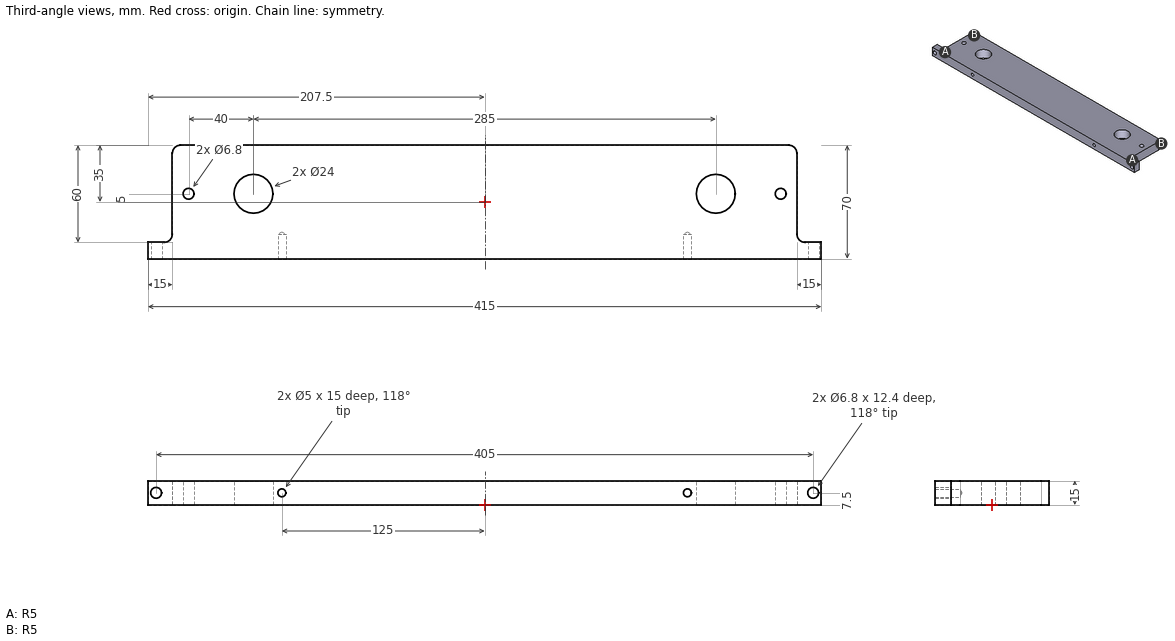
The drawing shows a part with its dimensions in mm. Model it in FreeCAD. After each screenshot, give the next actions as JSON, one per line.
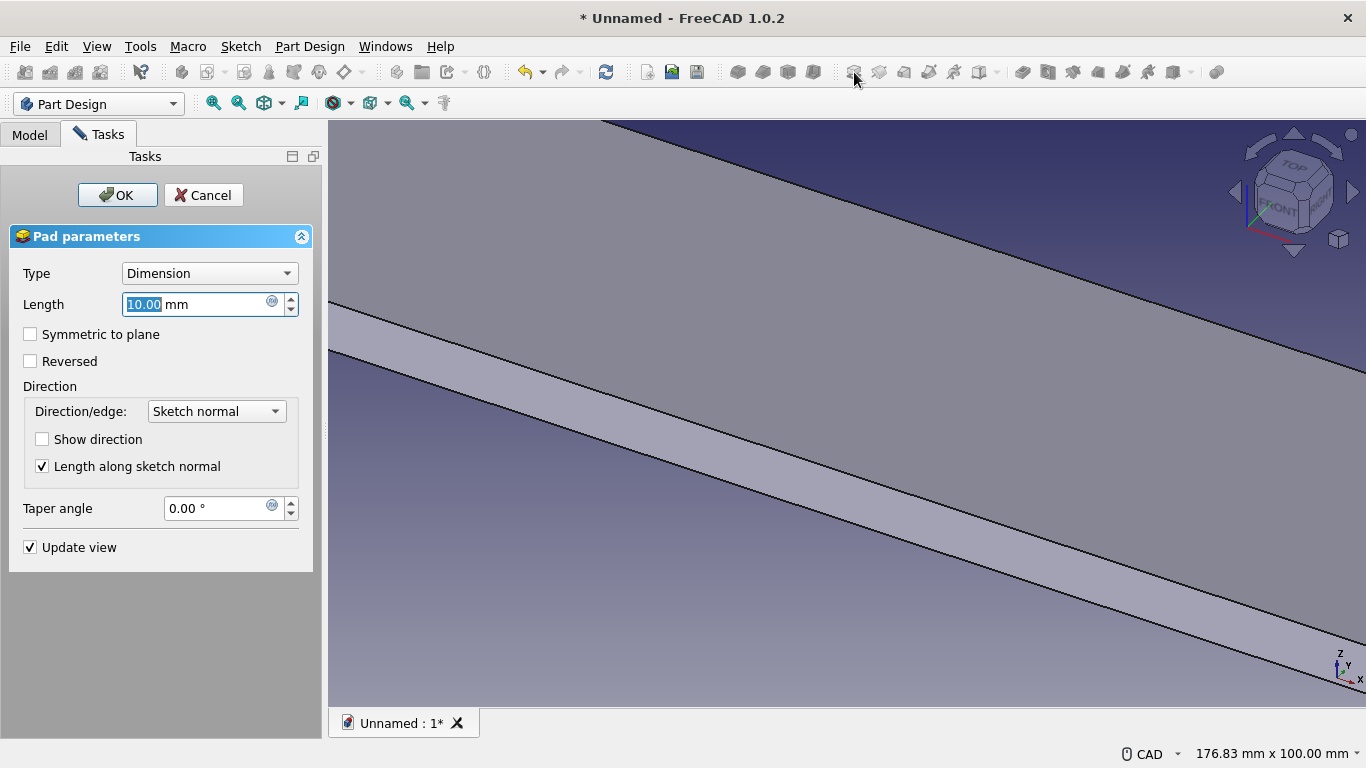
{"action": "type", "text": "15"}
{"action": "key", "text": "Tab"}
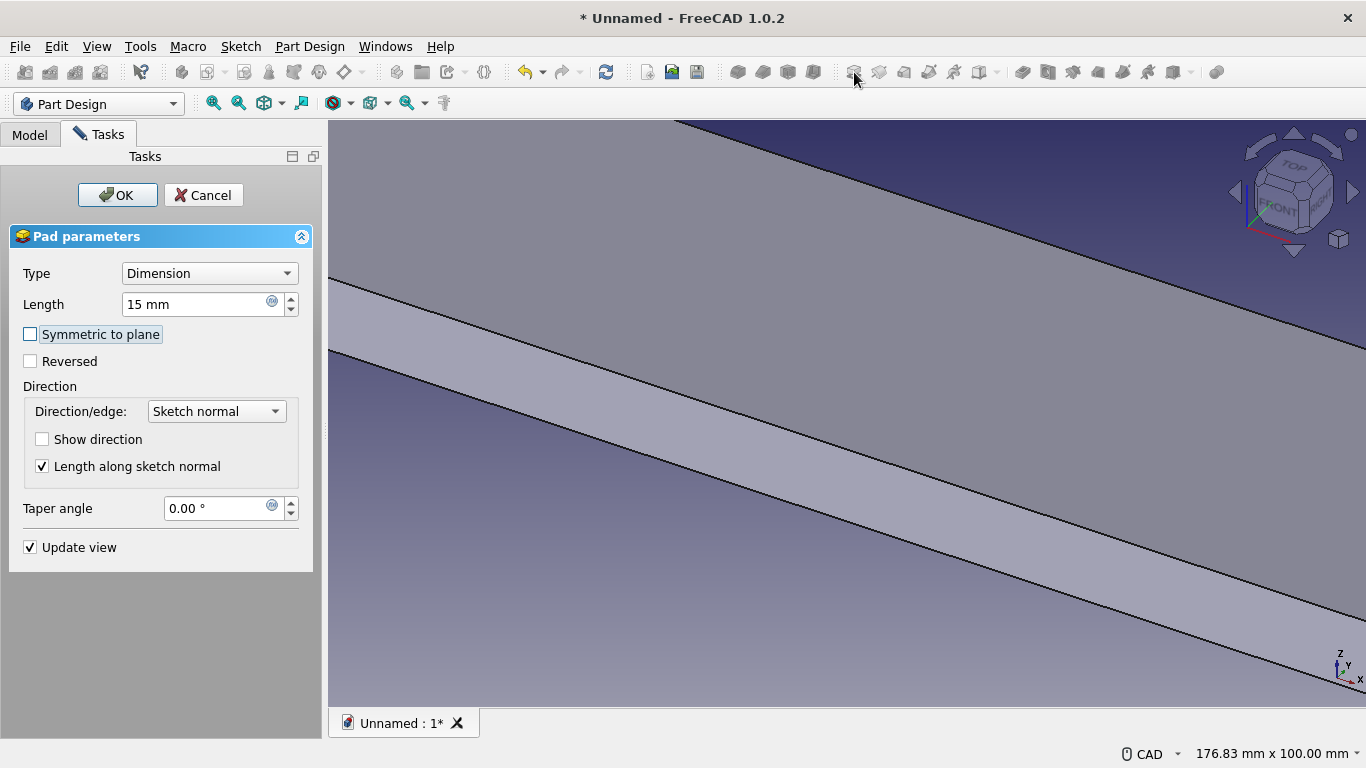
{"action": "left_click", "coordinate": [118, 195]}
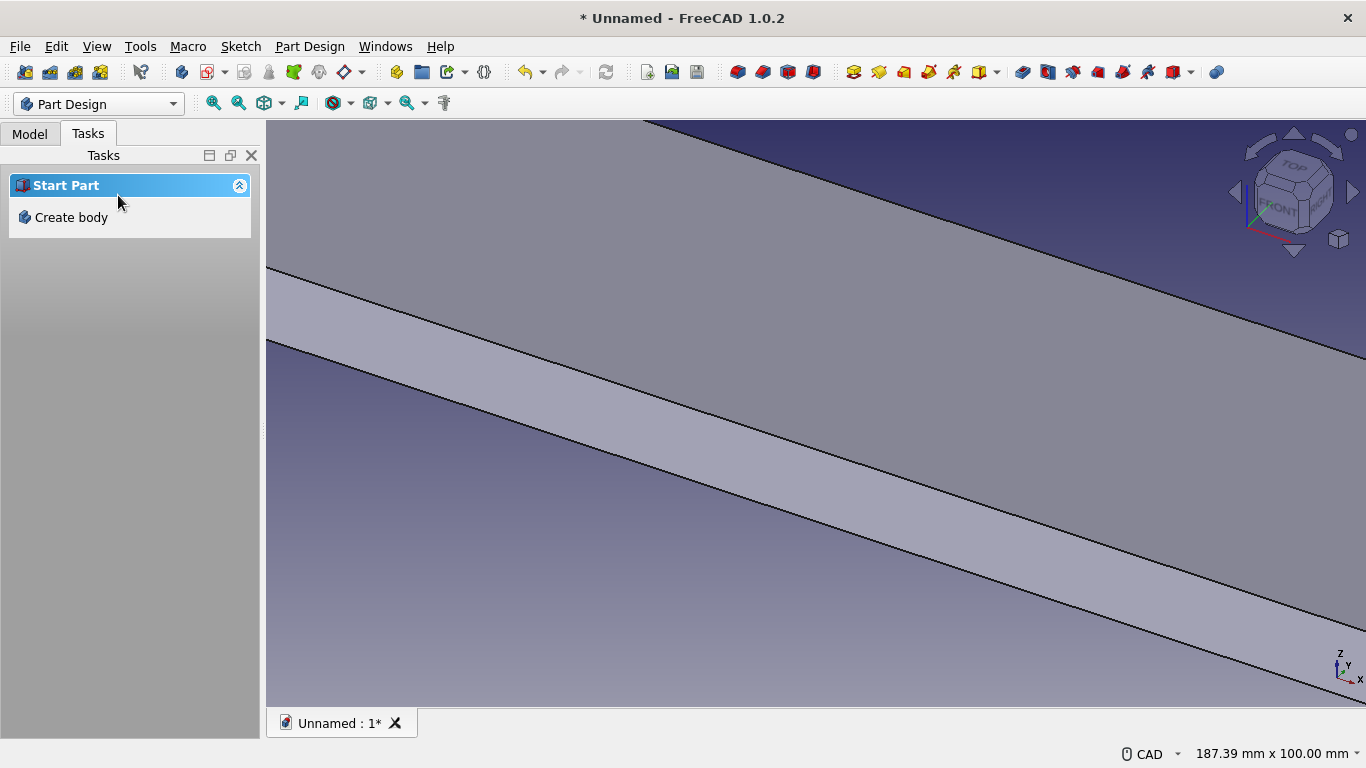
{"action": "key", "text": "v f"}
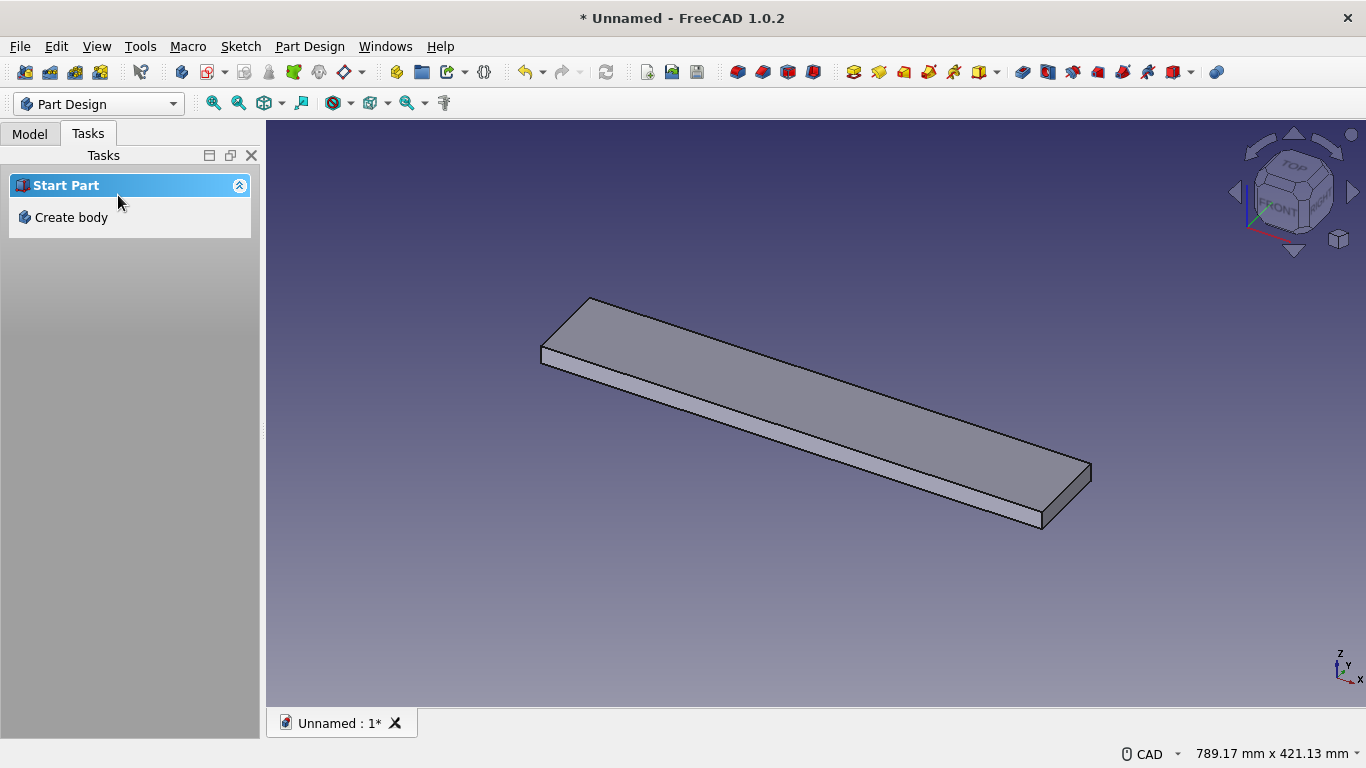
{"action": "left_click", "coordinate": [959, 451]}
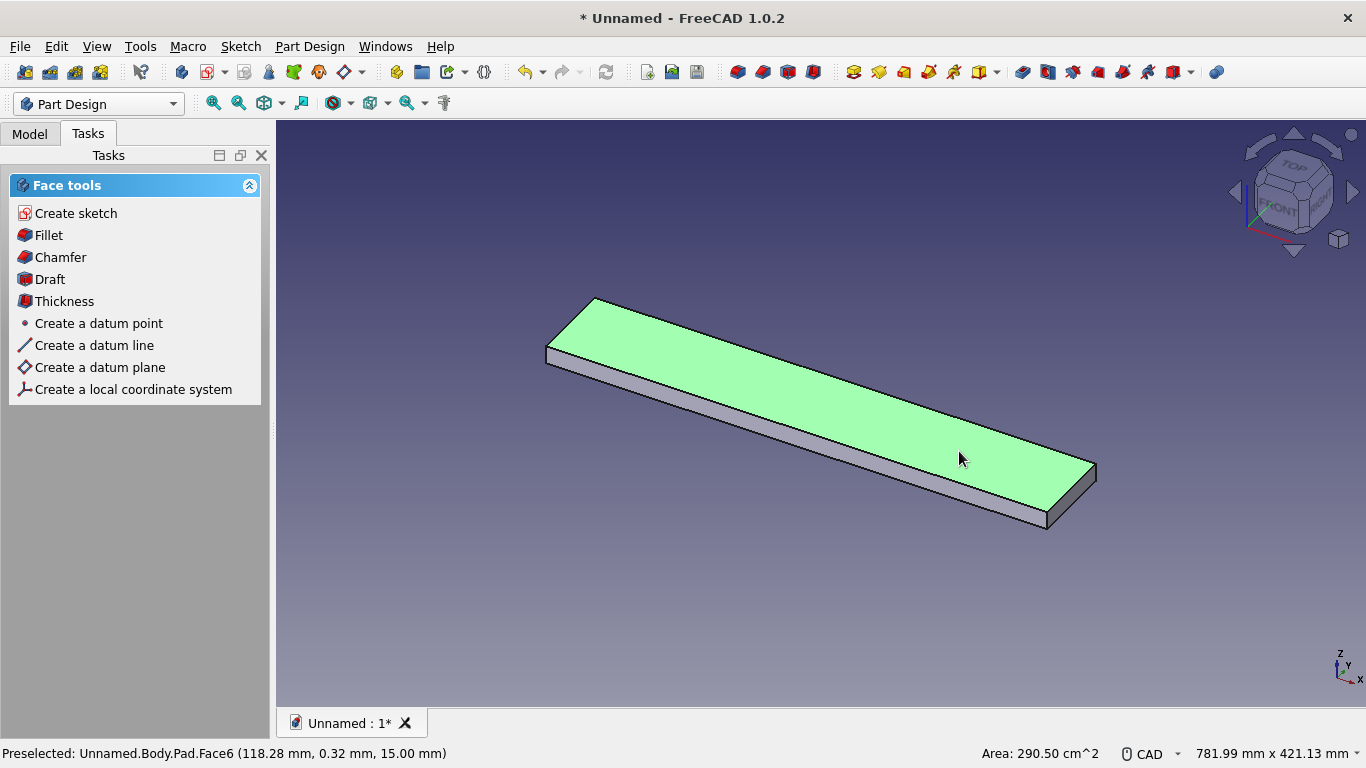
{"action": "left_click", "coordinate": [206, 72]}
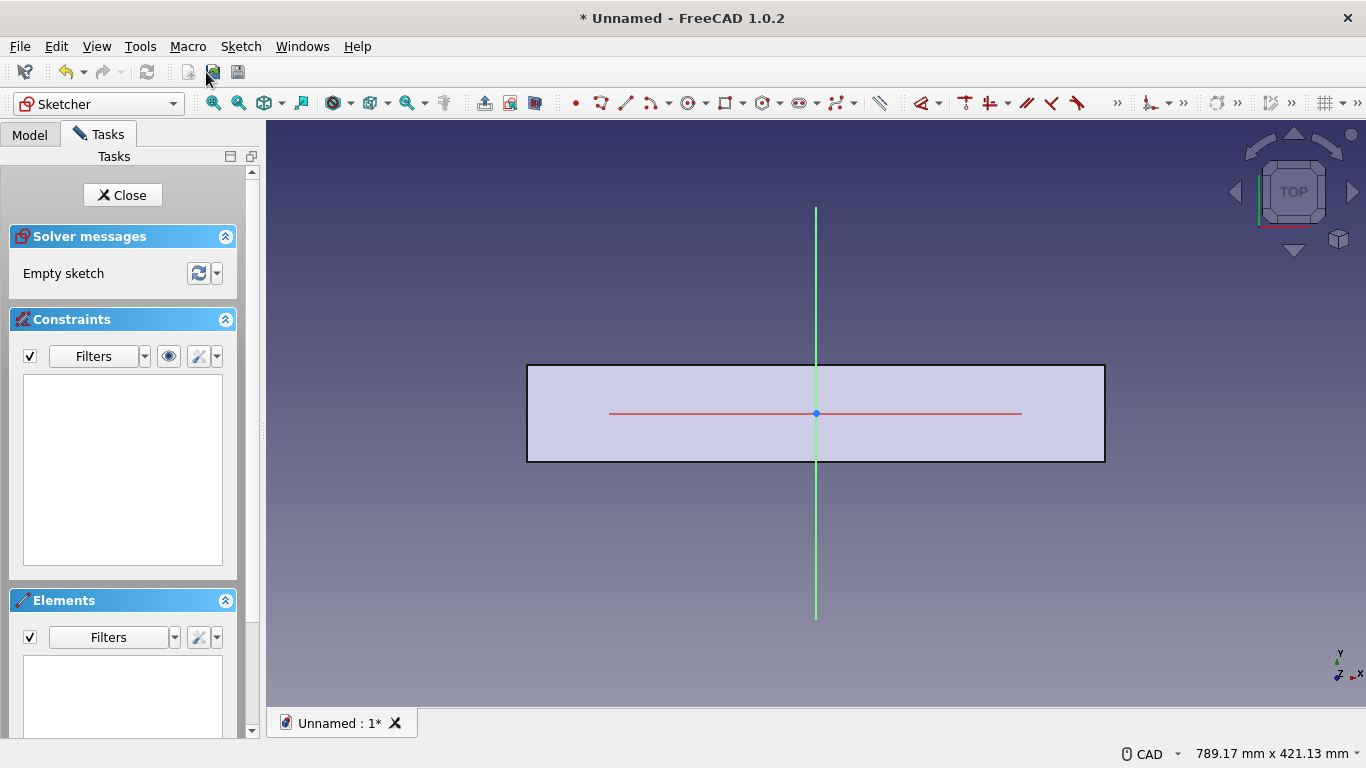
{"action": "key", "text": "g c"}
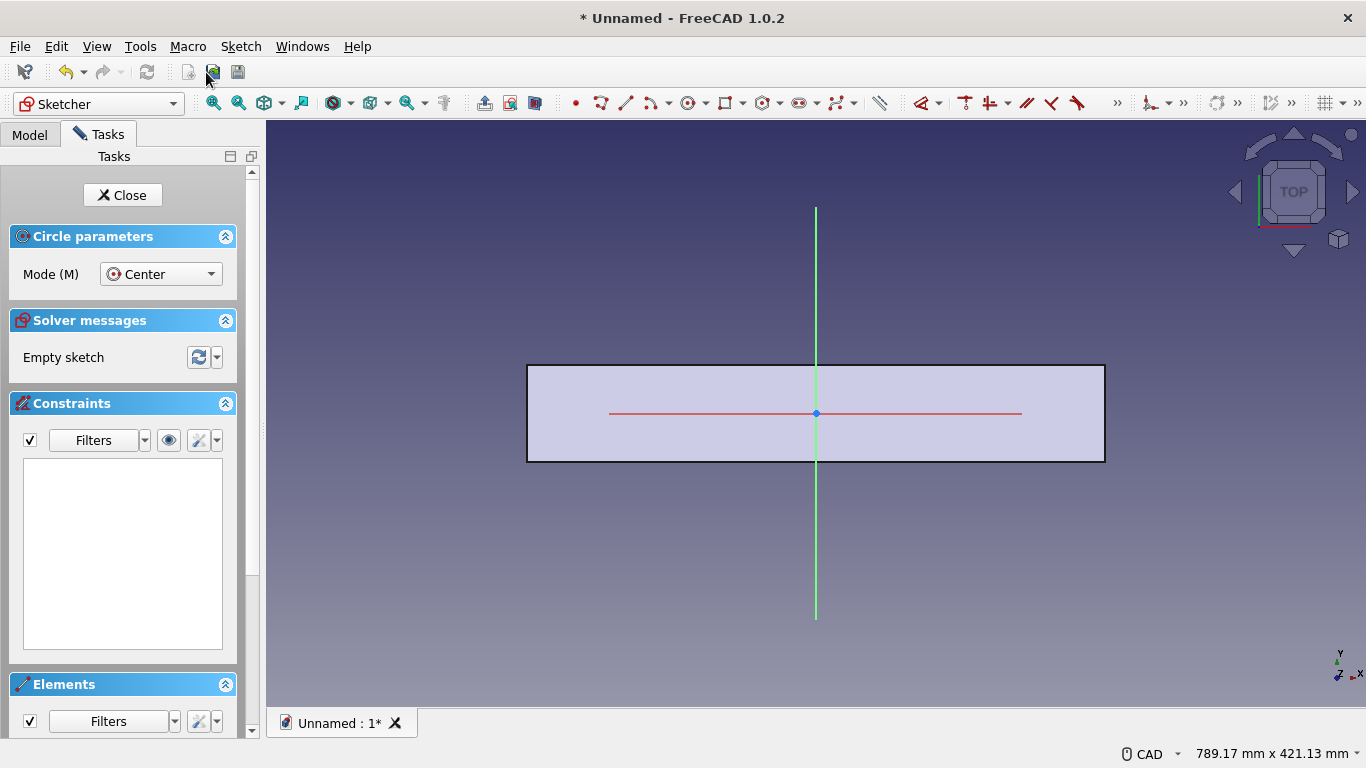
{"action": "scroll", "coordinate": [562, 407], "scroll_direction": "up", "scroll_amount": 8}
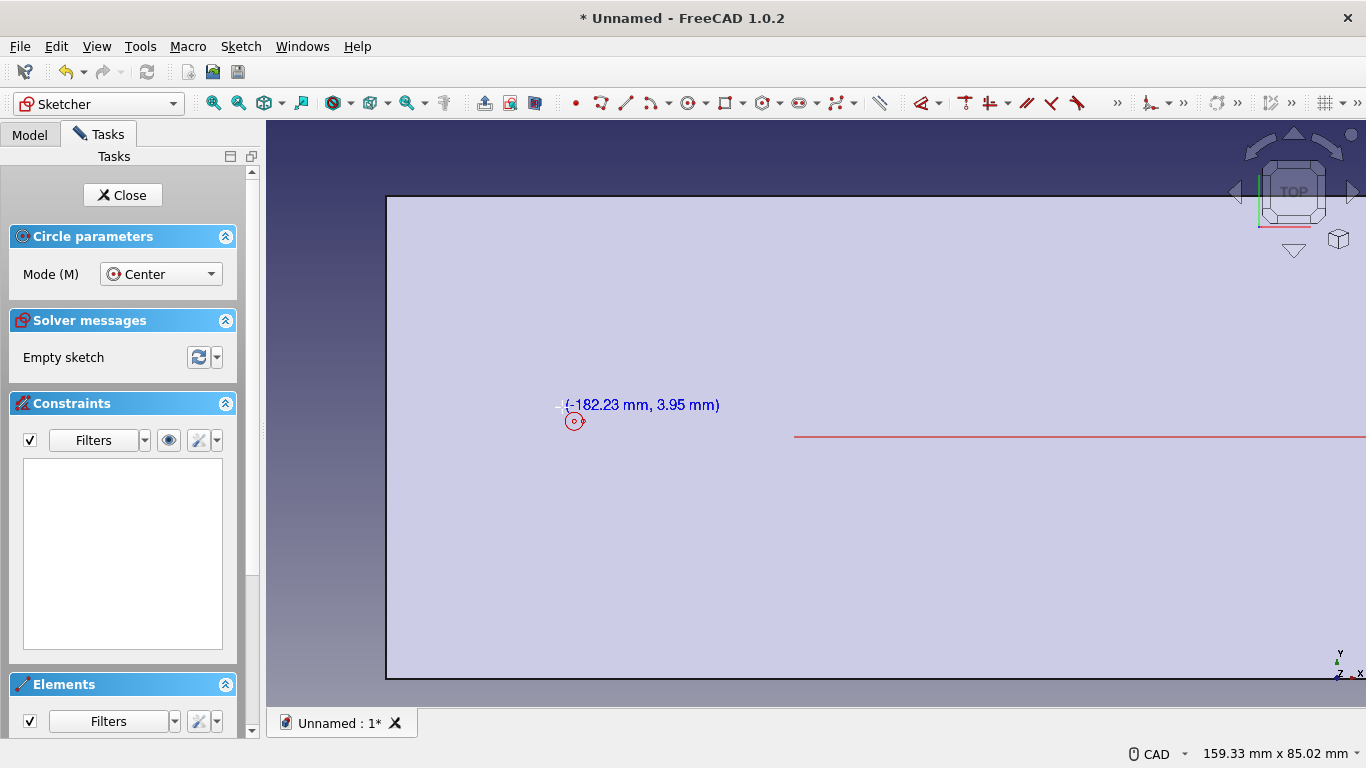
{"action": "left_click", "coordinate": [559, 403]}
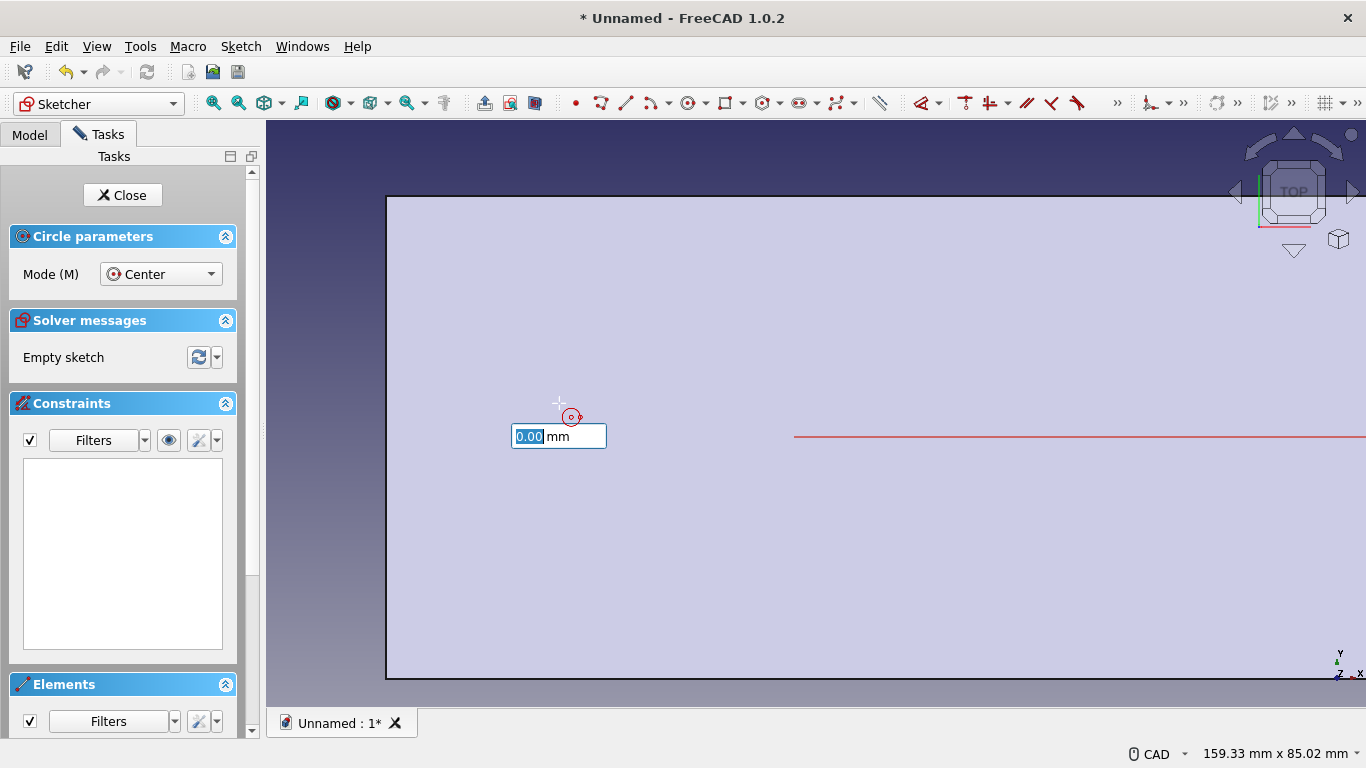
{"action": "scroll", "coordinate": [397, 417], "scroll_direction": "down", "scroll_amount": 7}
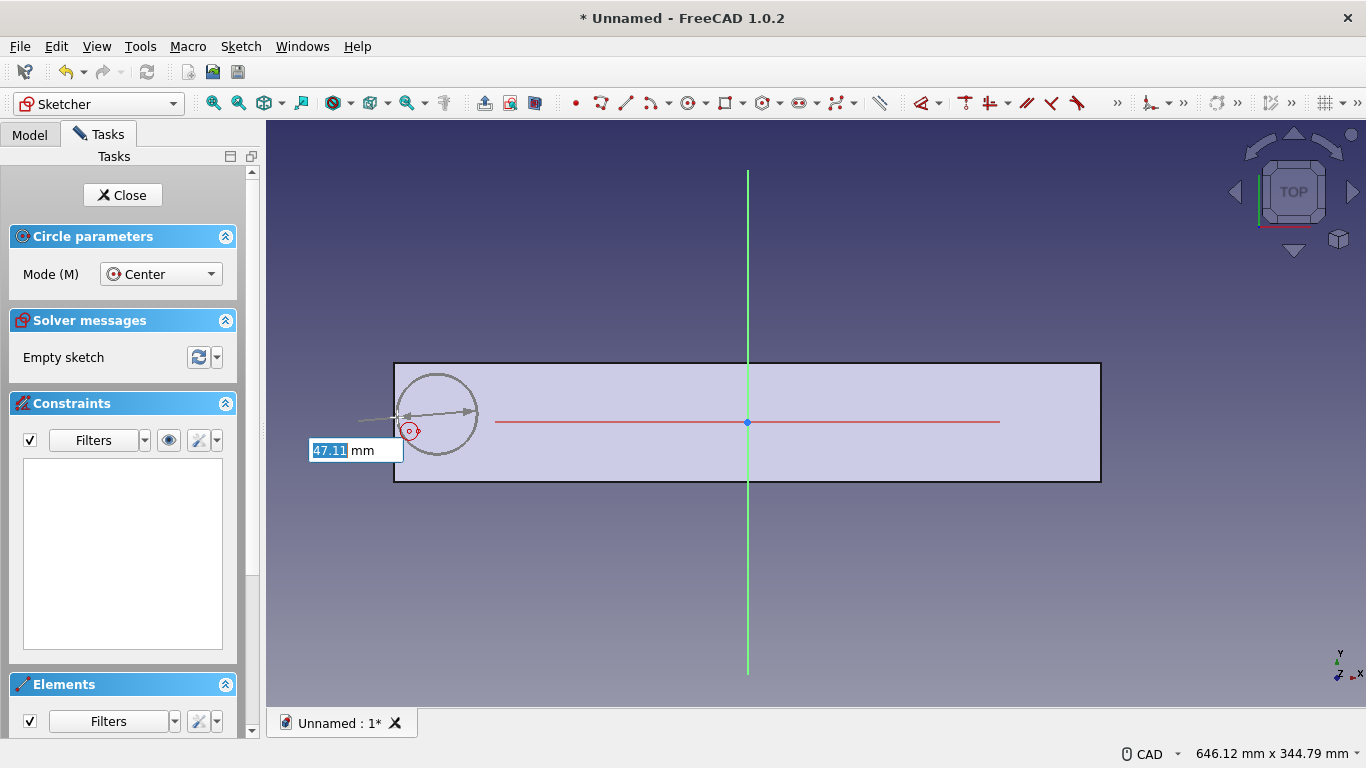
{"action": "scroll", "coordinate": [441, 410], "scroll_direction": "up", "scroll_amount": 2}
{"action": "mouse_move", "coordinate": [441, 409]}